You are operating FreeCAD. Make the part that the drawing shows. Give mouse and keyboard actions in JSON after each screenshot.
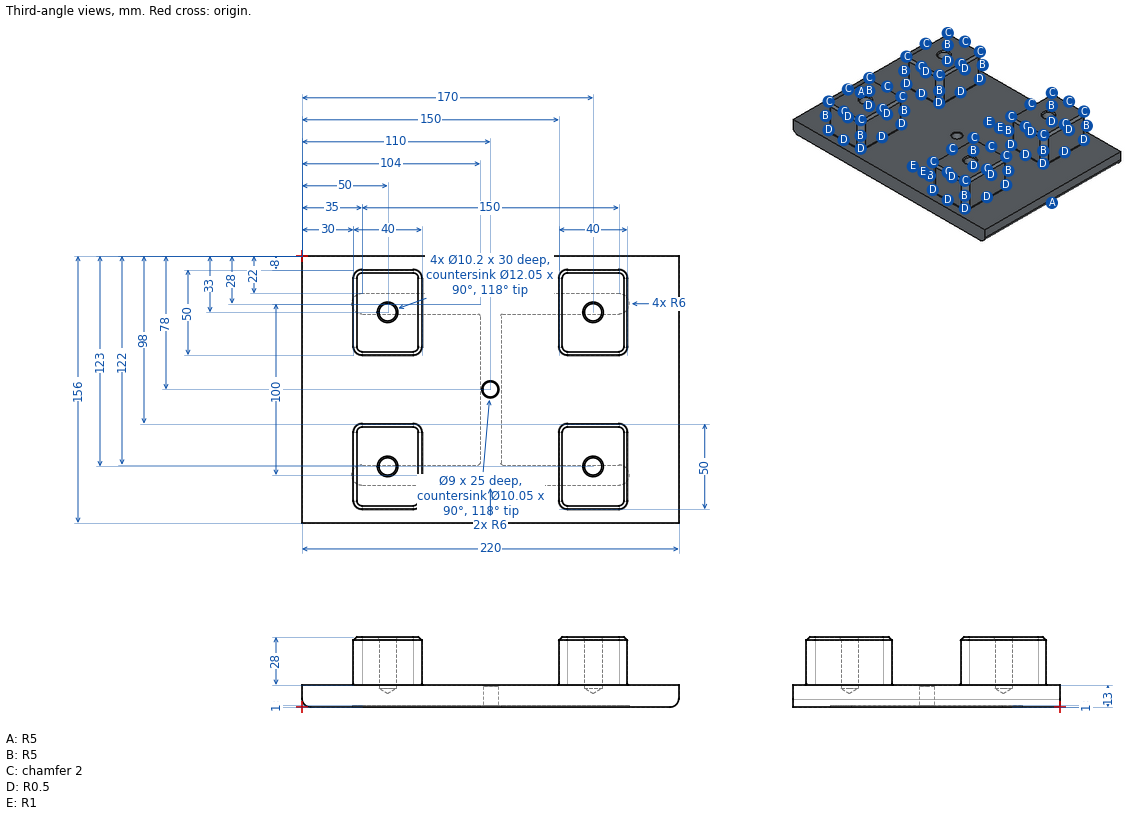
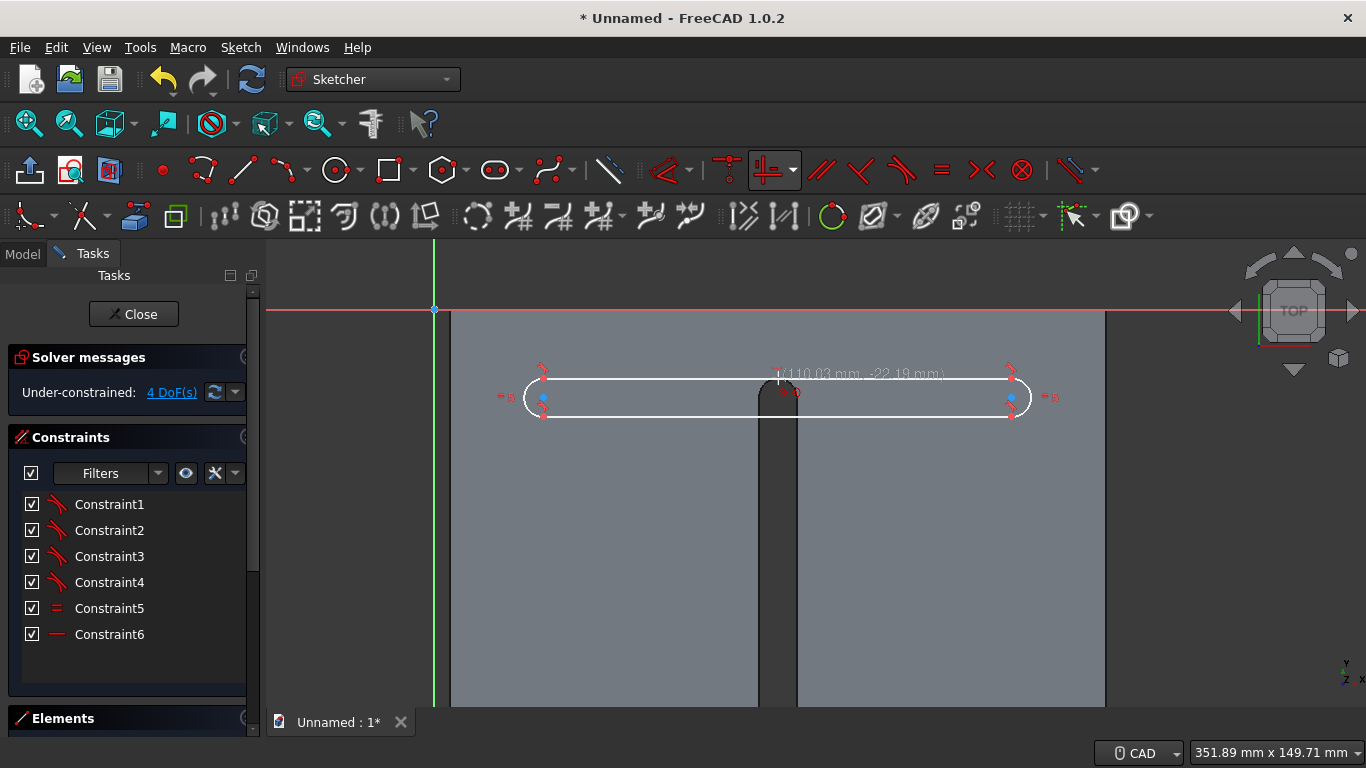
{"action": "scroll", "coordinate": [778, 379], "scroll_direction": "down", "scroll_amount": 2}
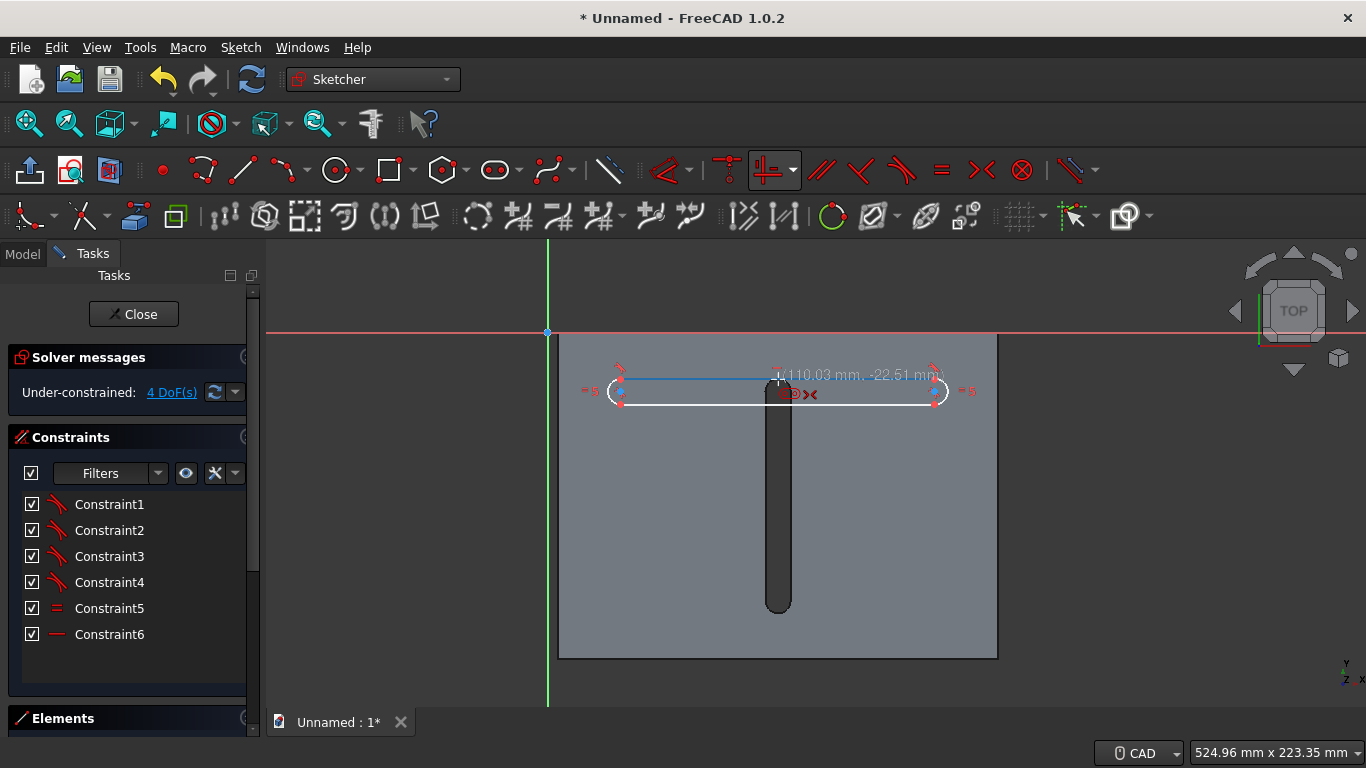
{"action": "scroll", "coordinate": [621, 601], "scroll_direction": "up", "scroll_amount": 3}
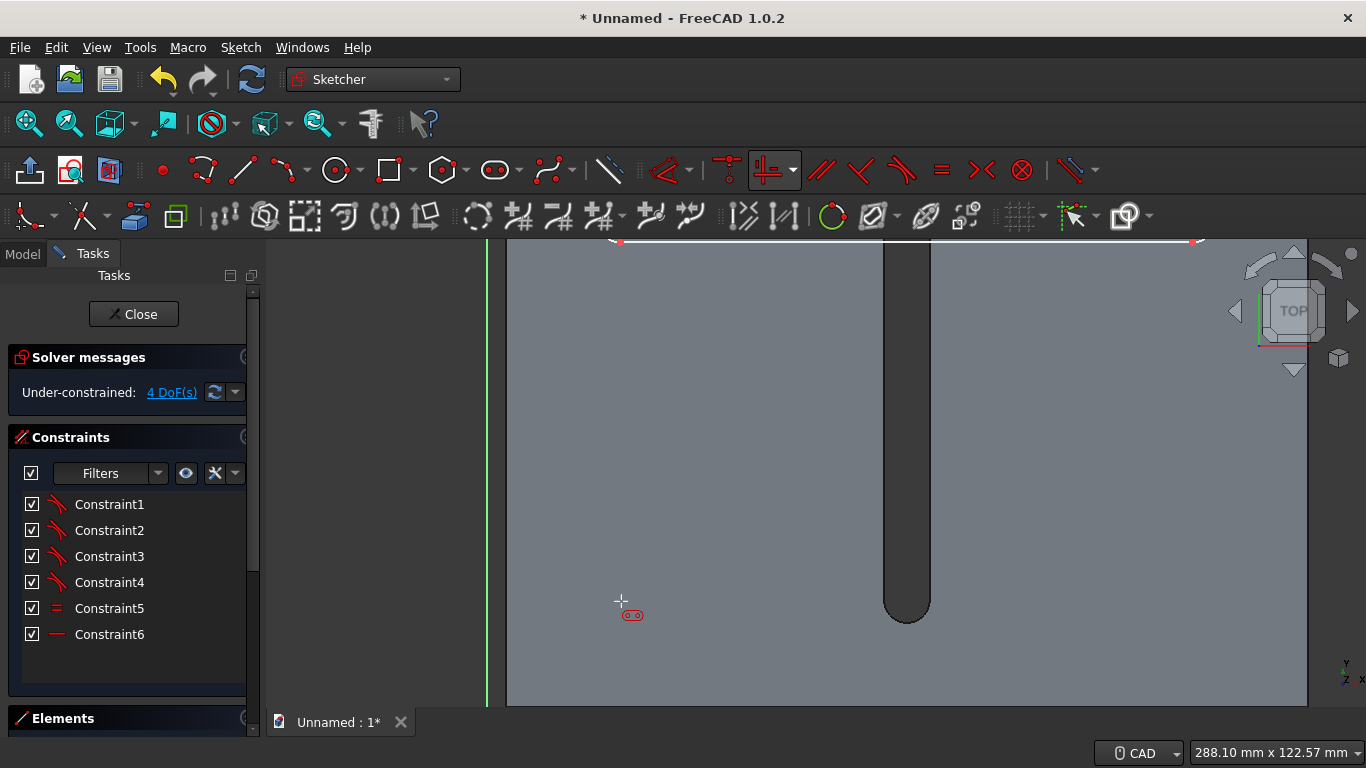
{"action": "left_click", "coordinate": [621, 600]}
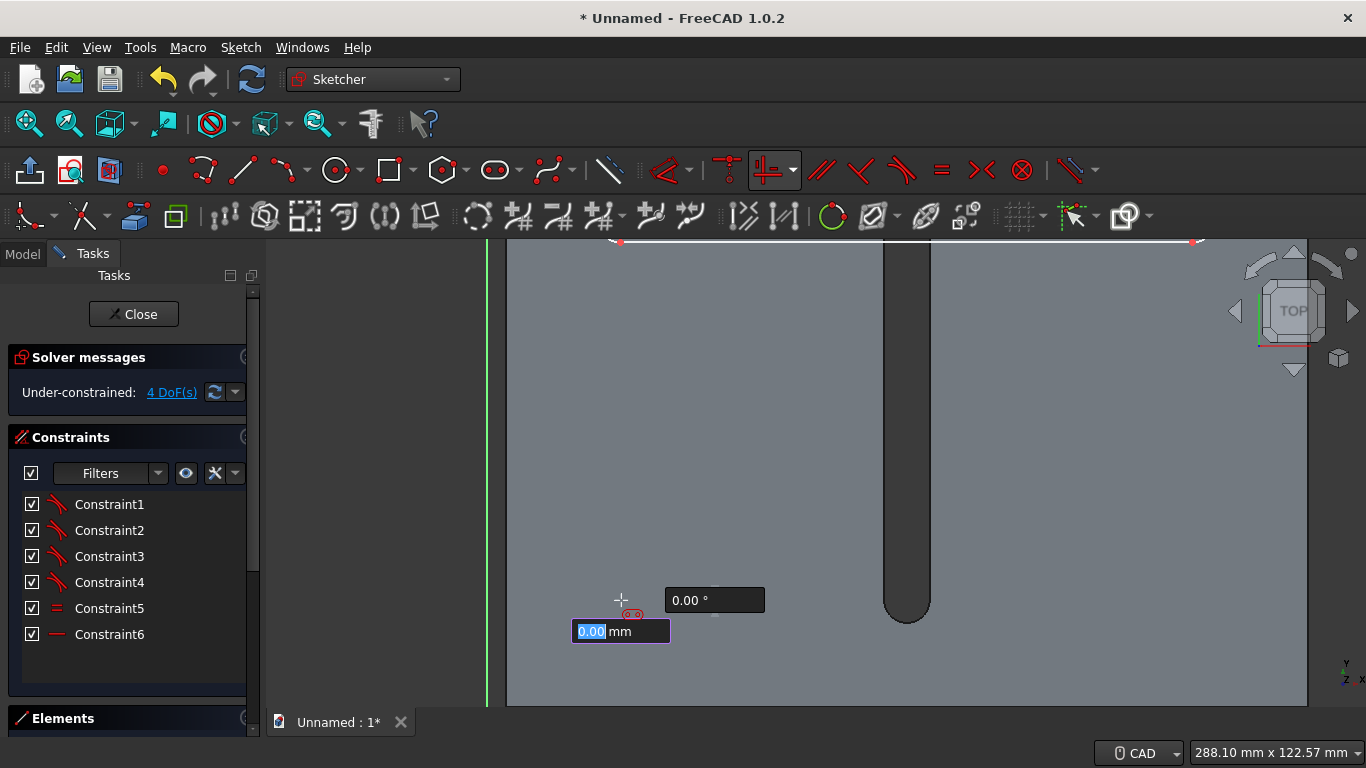
{"action": "left_click", "coordinate": [1193, 600]}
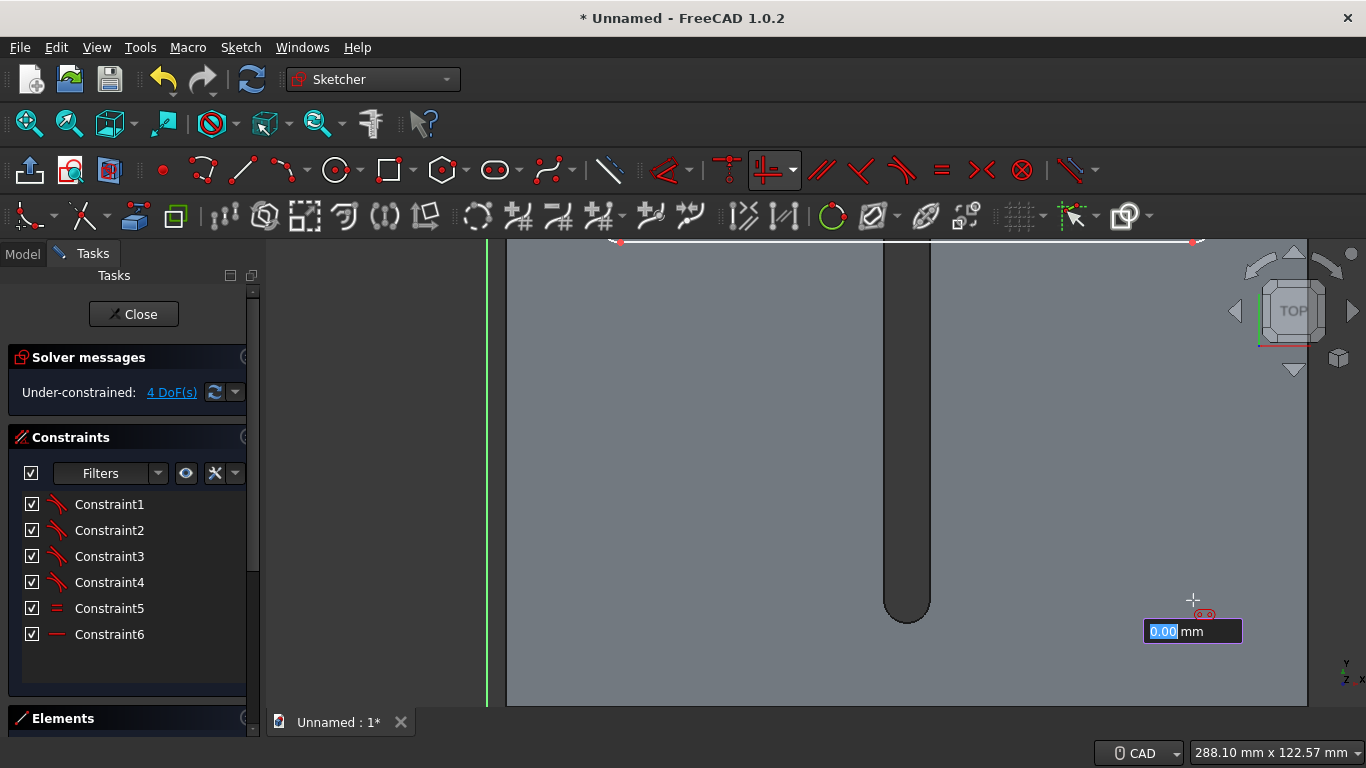
{"action": "left_click", "coordinate": [907, 623]}
{"action": "key", "text": "Escape"}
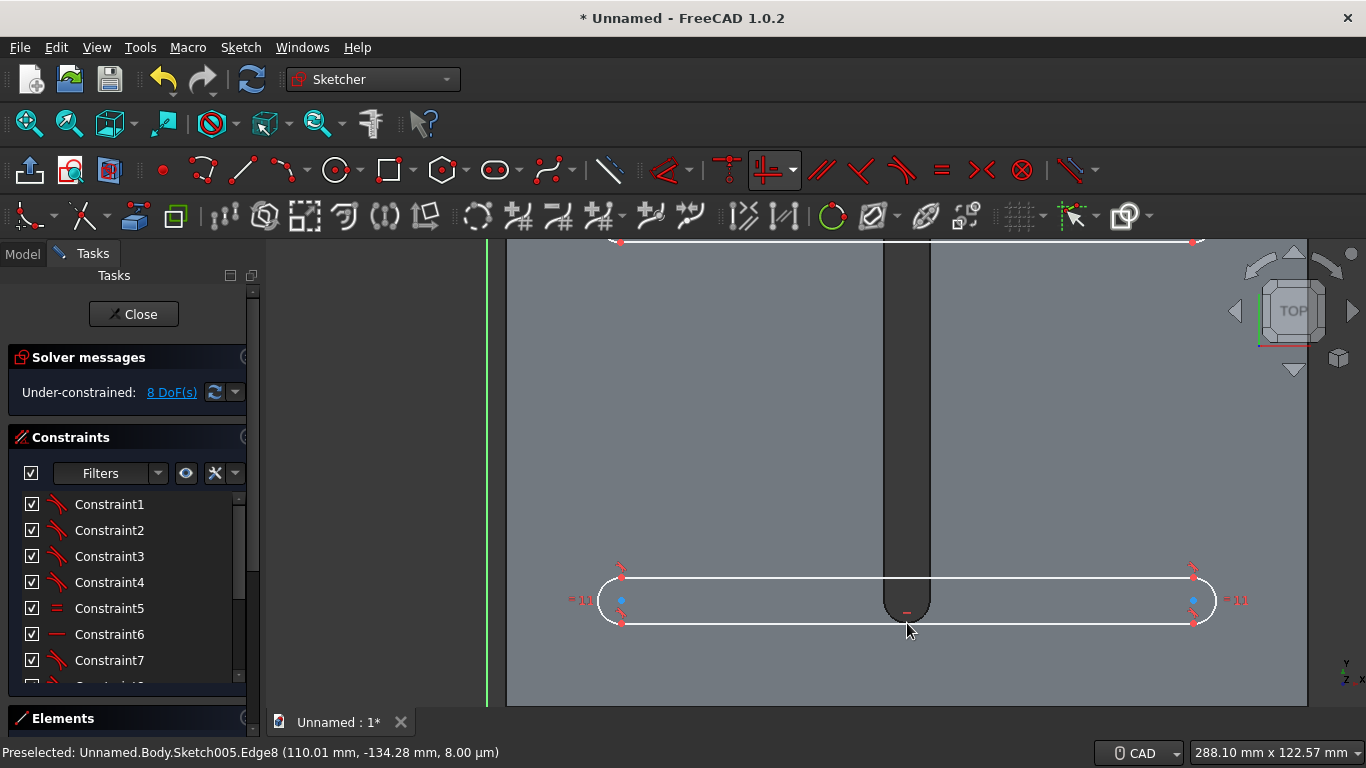
{"action": "scroll", "coordinate": [621, 602], "scroll_direction": "down", "scroll_amount": 3}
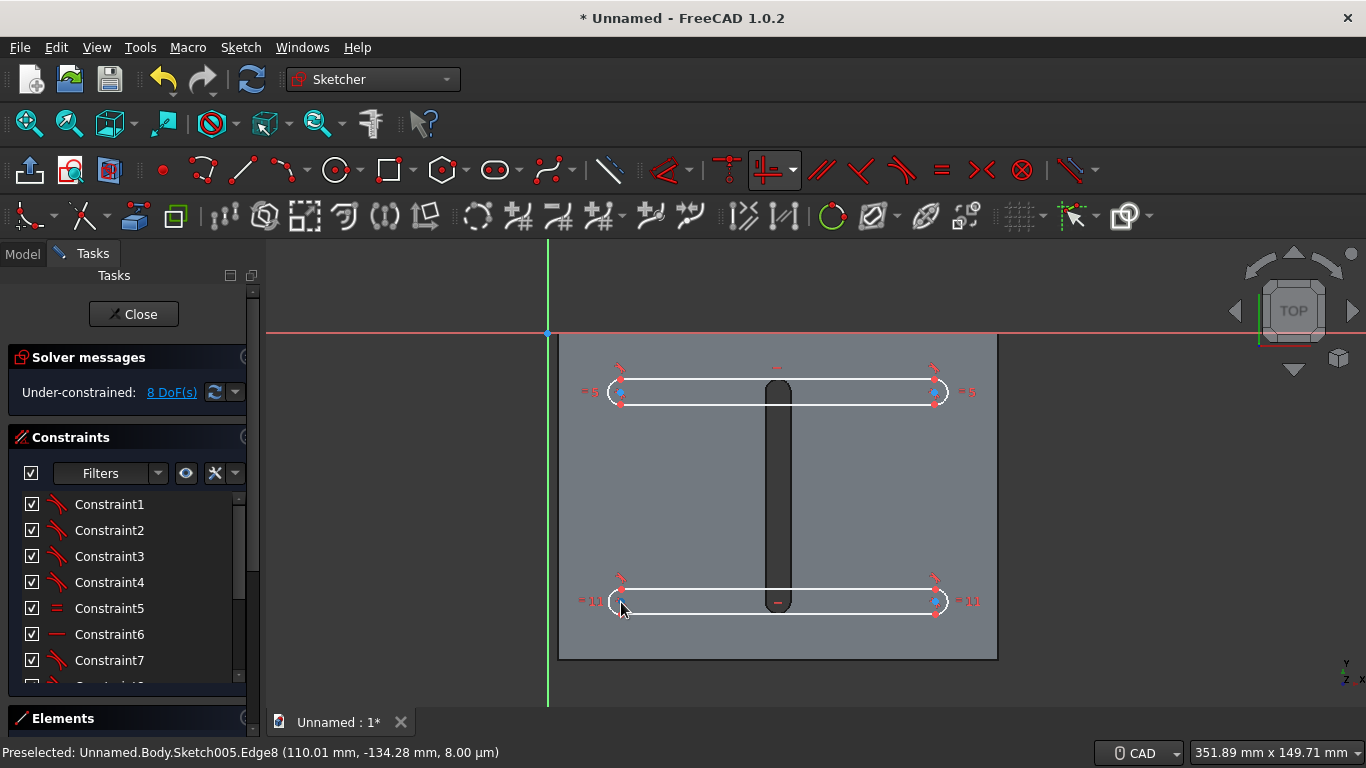
{"action": "left_click", "coordinate": [610, 385]}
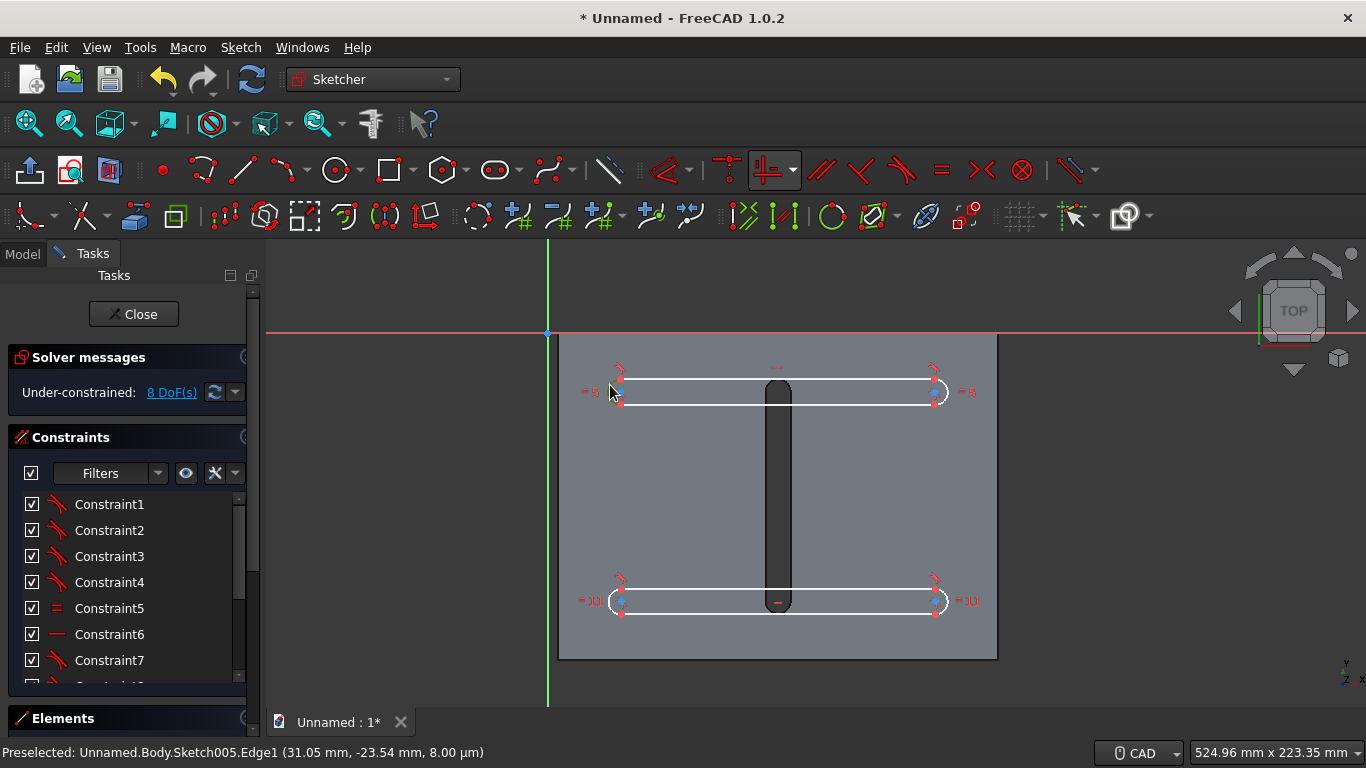
{"action": "left_click", "coordinate": [611, 594]}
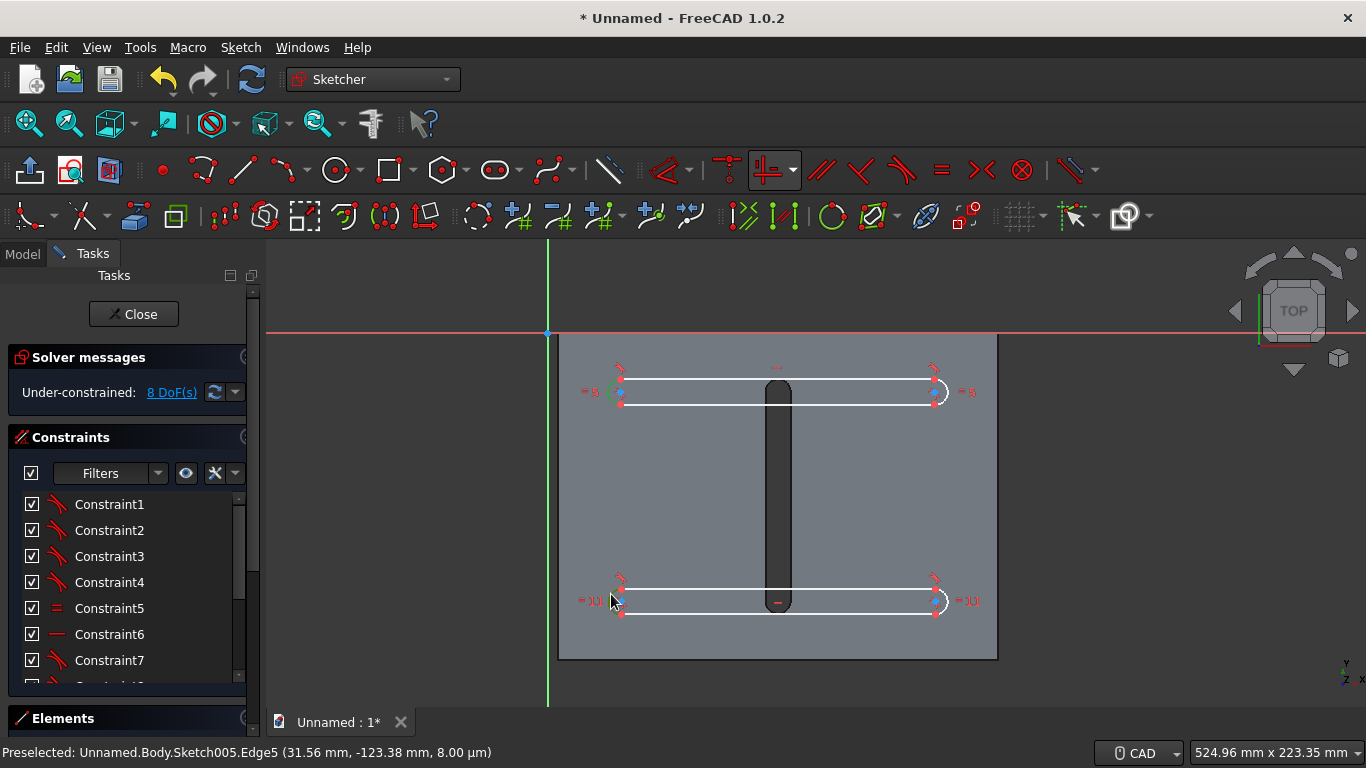
{"action": "key", "text": "e"}